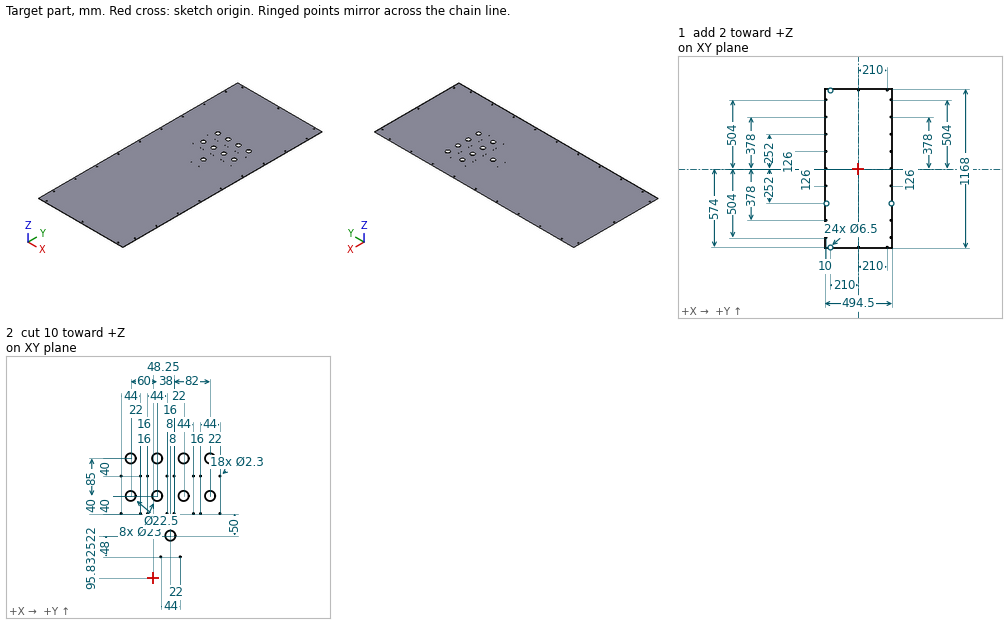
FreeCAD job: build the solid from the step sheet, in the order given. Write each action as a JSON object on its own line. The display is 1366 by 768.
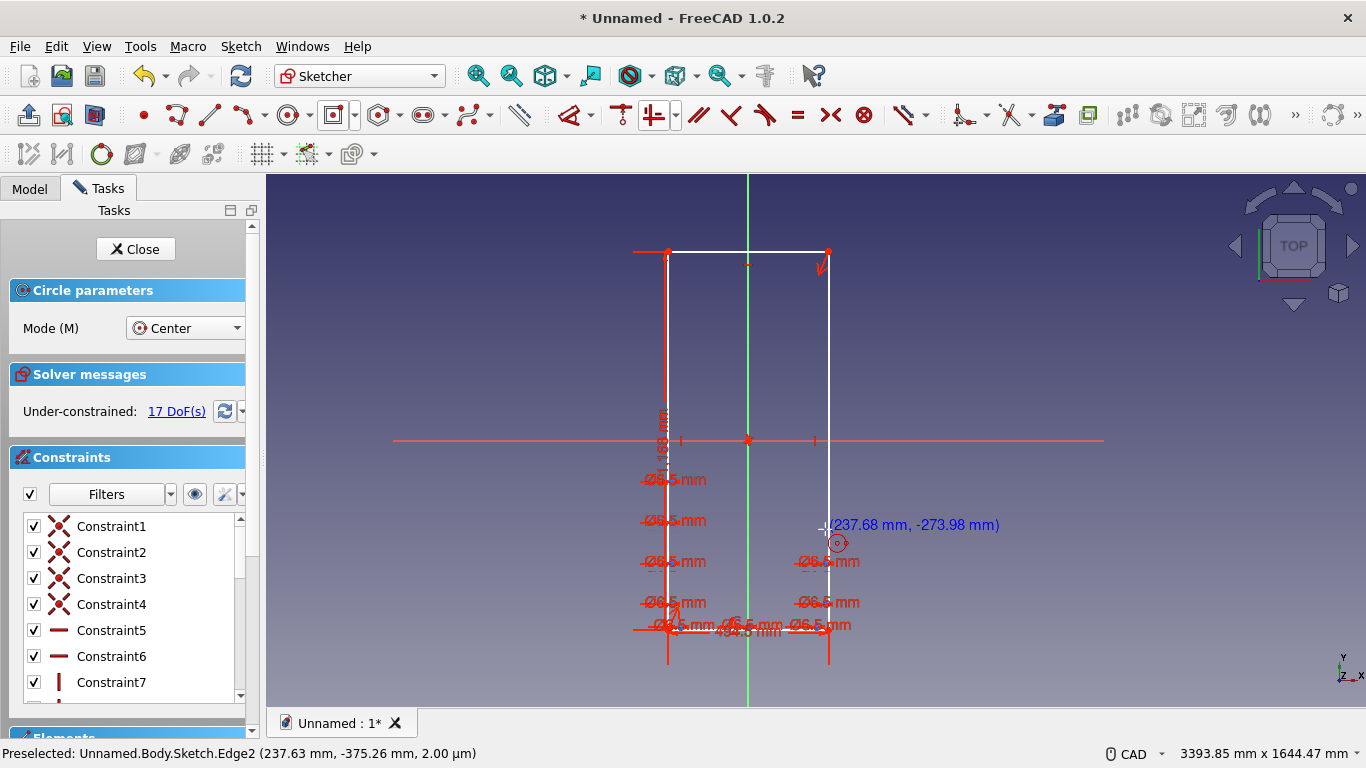
{"action": "scroll", "coordinate": [825, 523], "scroll_direction": "up", "scroll_amount": 8}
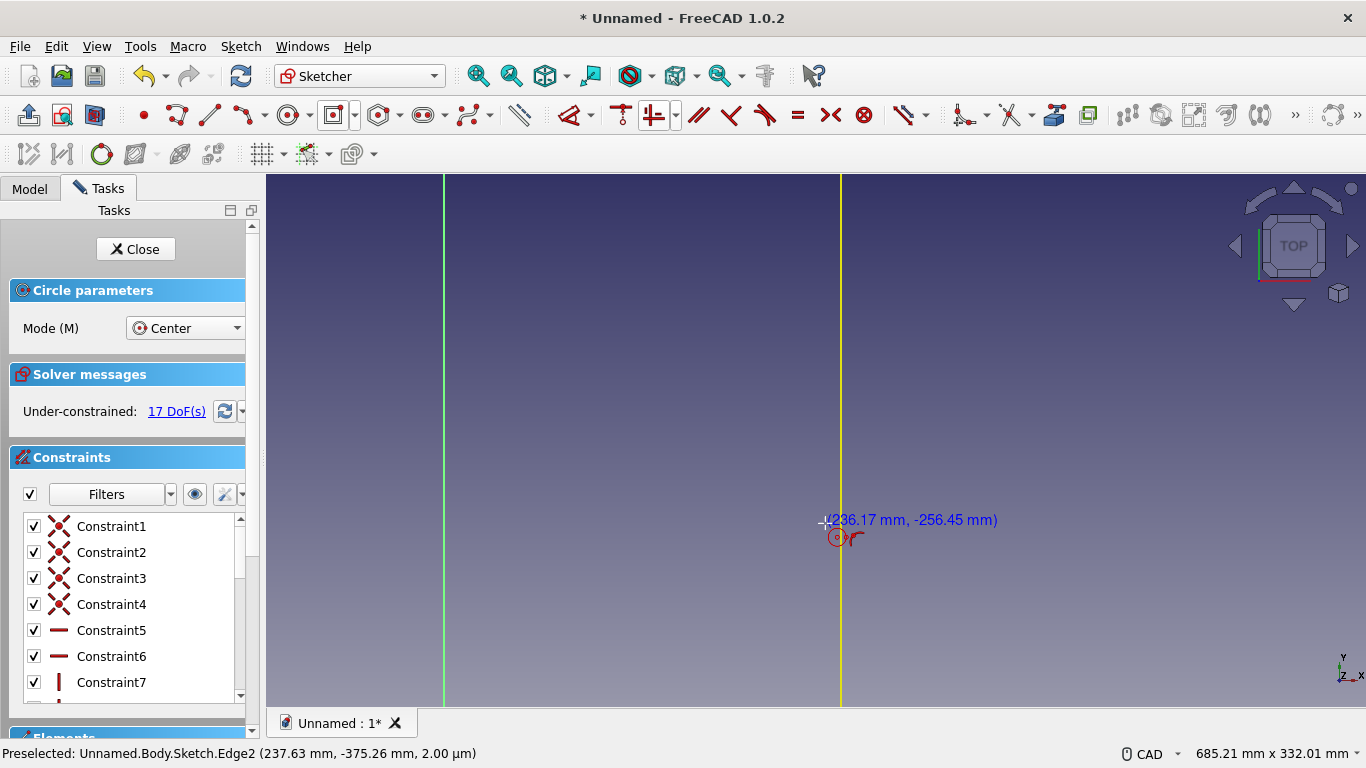
{"action": "left_click", "coordinate": [825, 518]}
{"action": "mouse_move", "coordinate": [821, 515]}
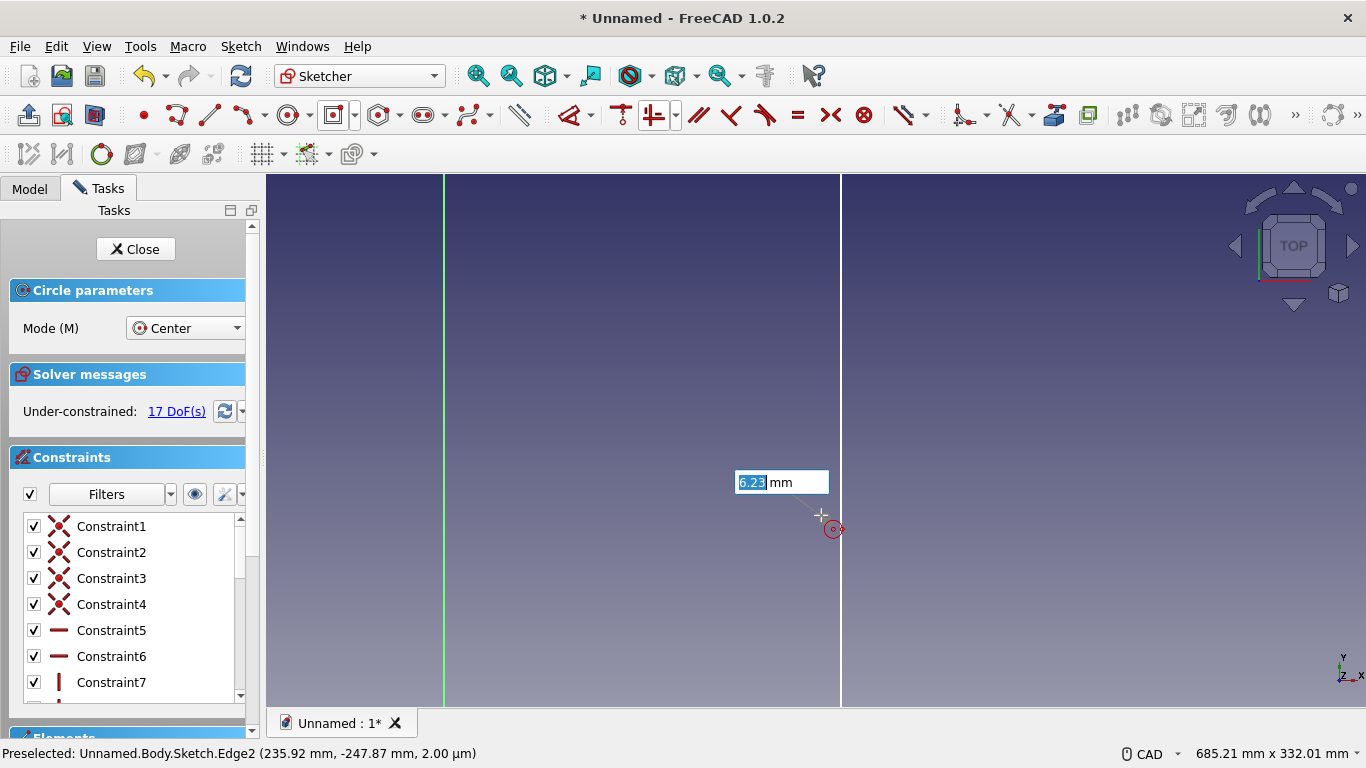
{"action": "type", "text": "6.5"}
{"action": "key", "text": "Return"}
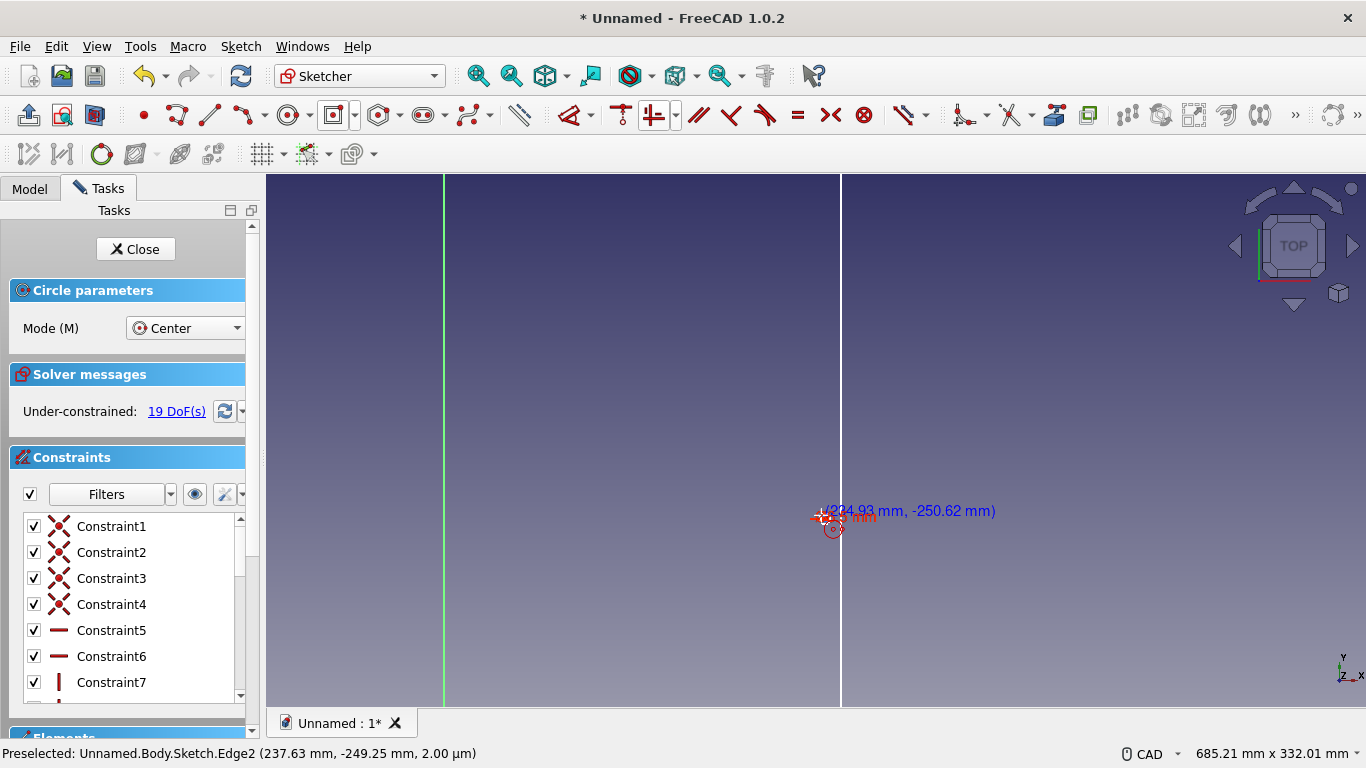
{"action": "scroll", "coordinate": [825, 316], "scroll_direction": "up", "scroll_amount": 8}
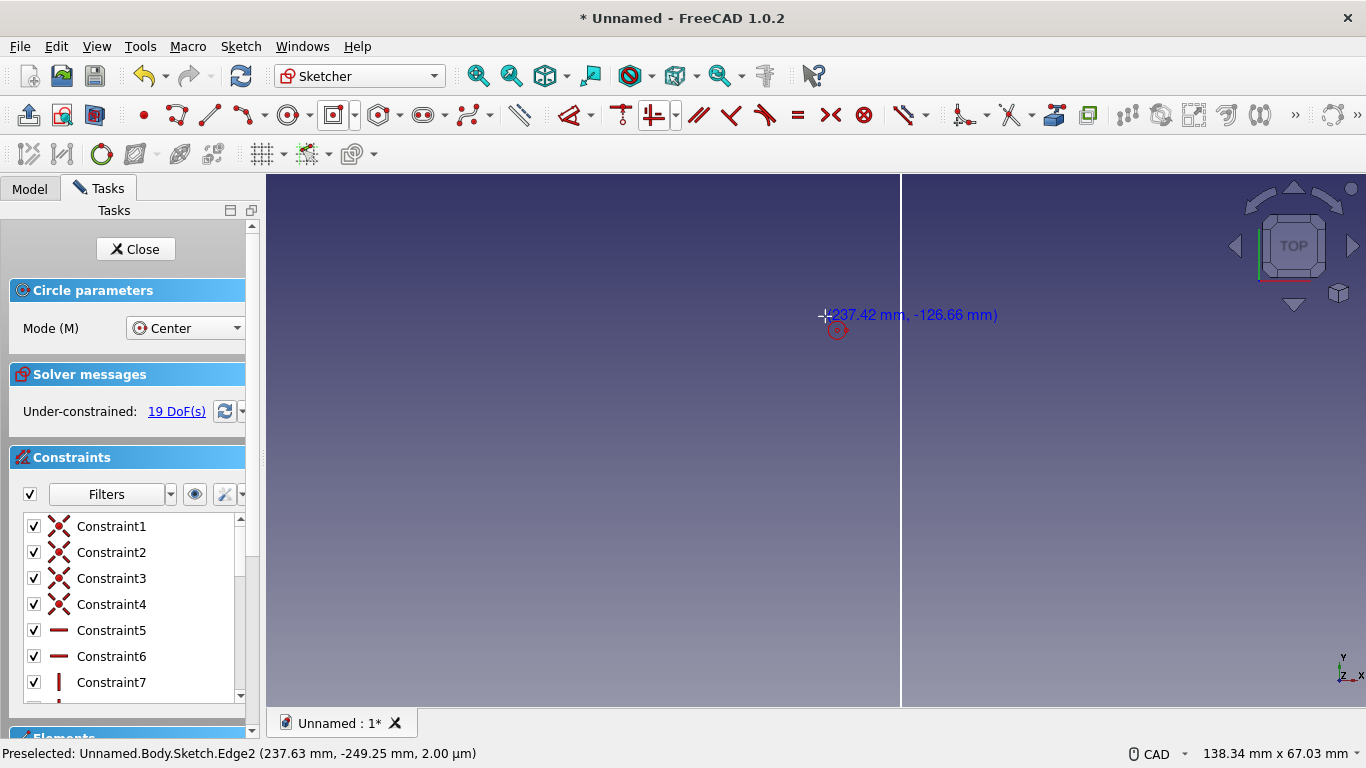
{"action": "scroll", "coordinate": [825, 488], "scroll_direction": "down", "scroll_amount": 16}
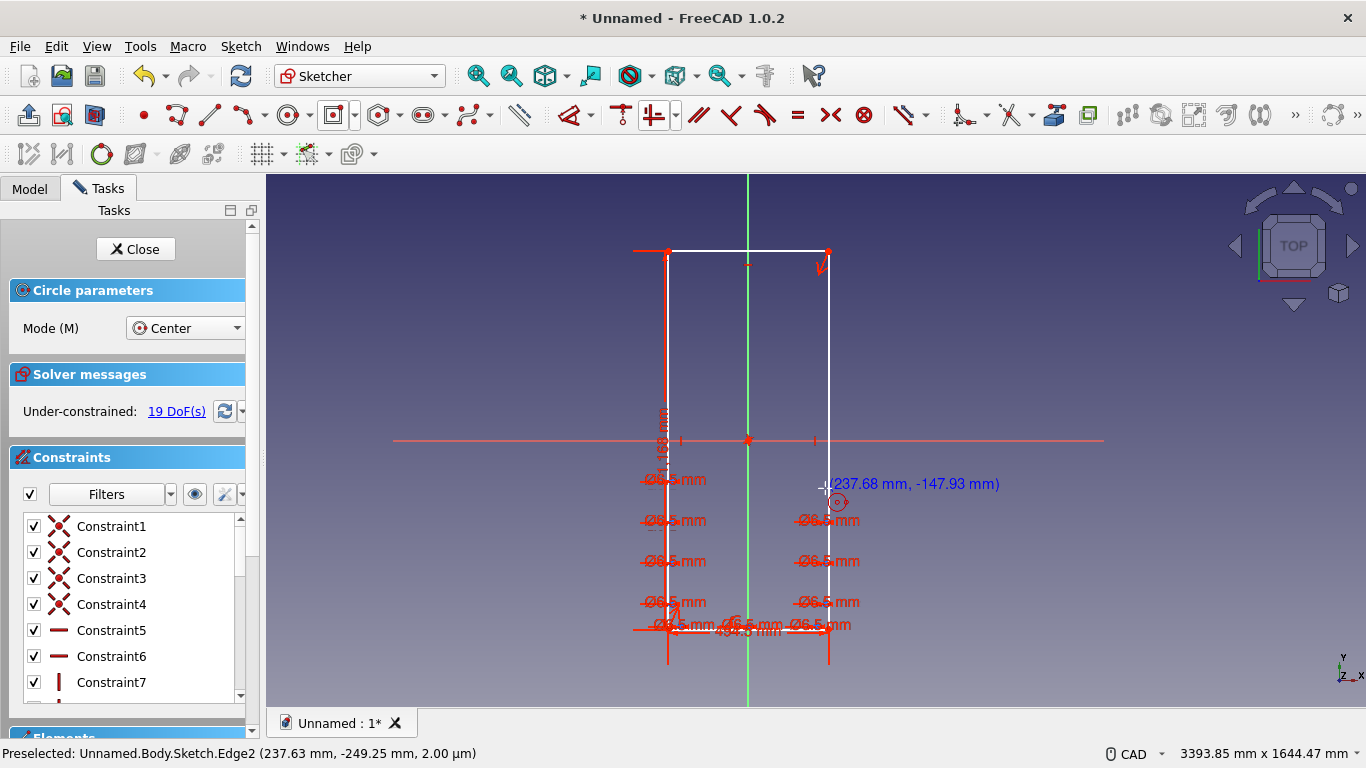
{"action": "scroll", "coordinate": [825, 481], "scroll_direction": "up", "scroll_amount": 8}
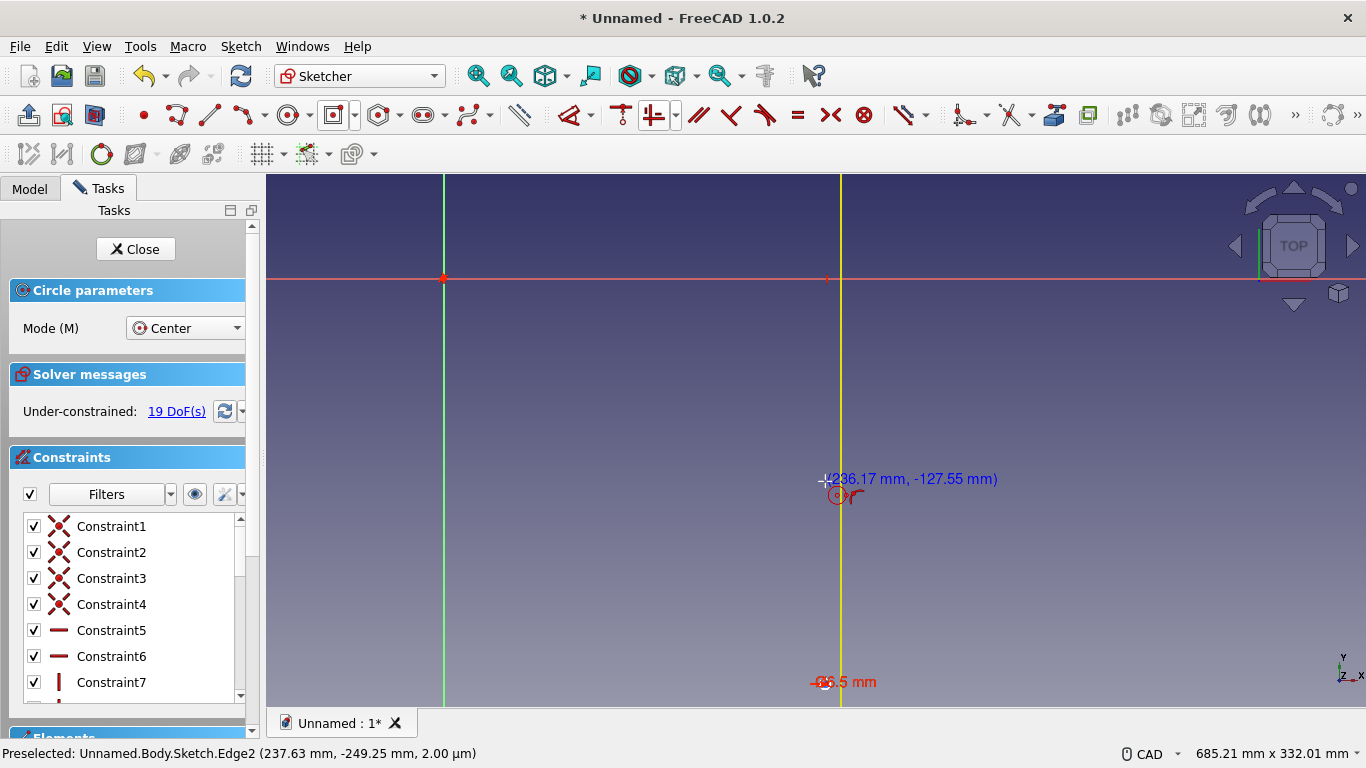
{"action": "left_click", "coordinate": [825, 481]}
{"action": "mouse_move", "coordinate": [821, 477]}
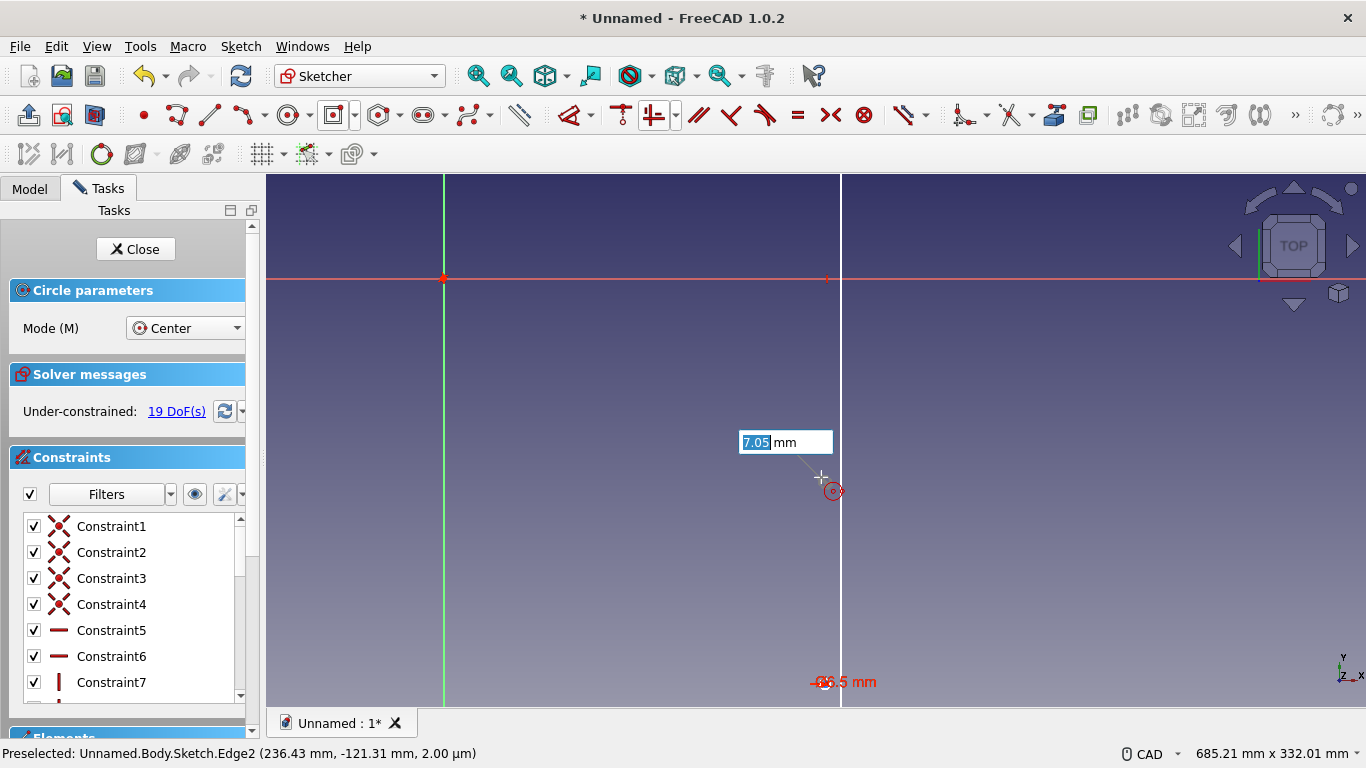
{"action": "type", "text": "6.5"}
{"action": "key", "text": "Return"}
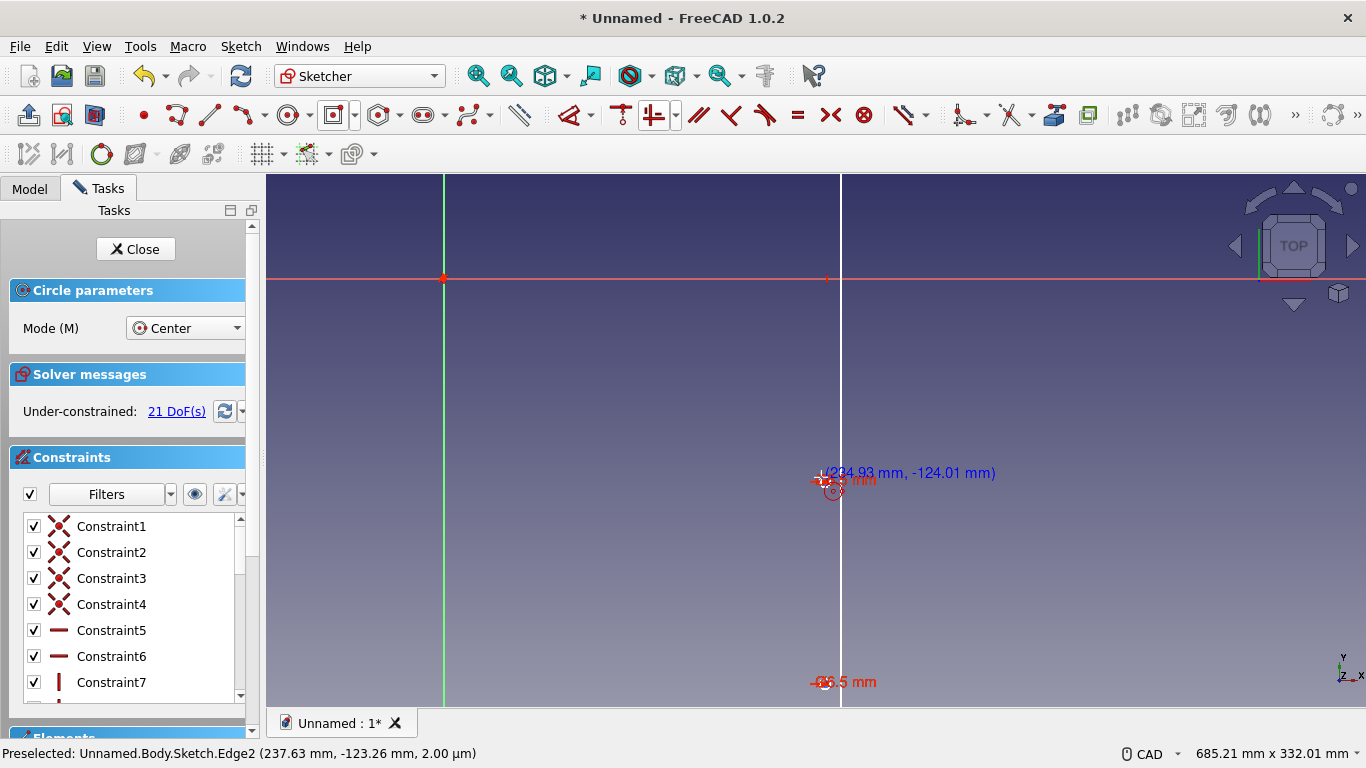
{"action": "scroll", "coordinate": [808, 472], "scroll_direction": "down", "scroll_amount": 9}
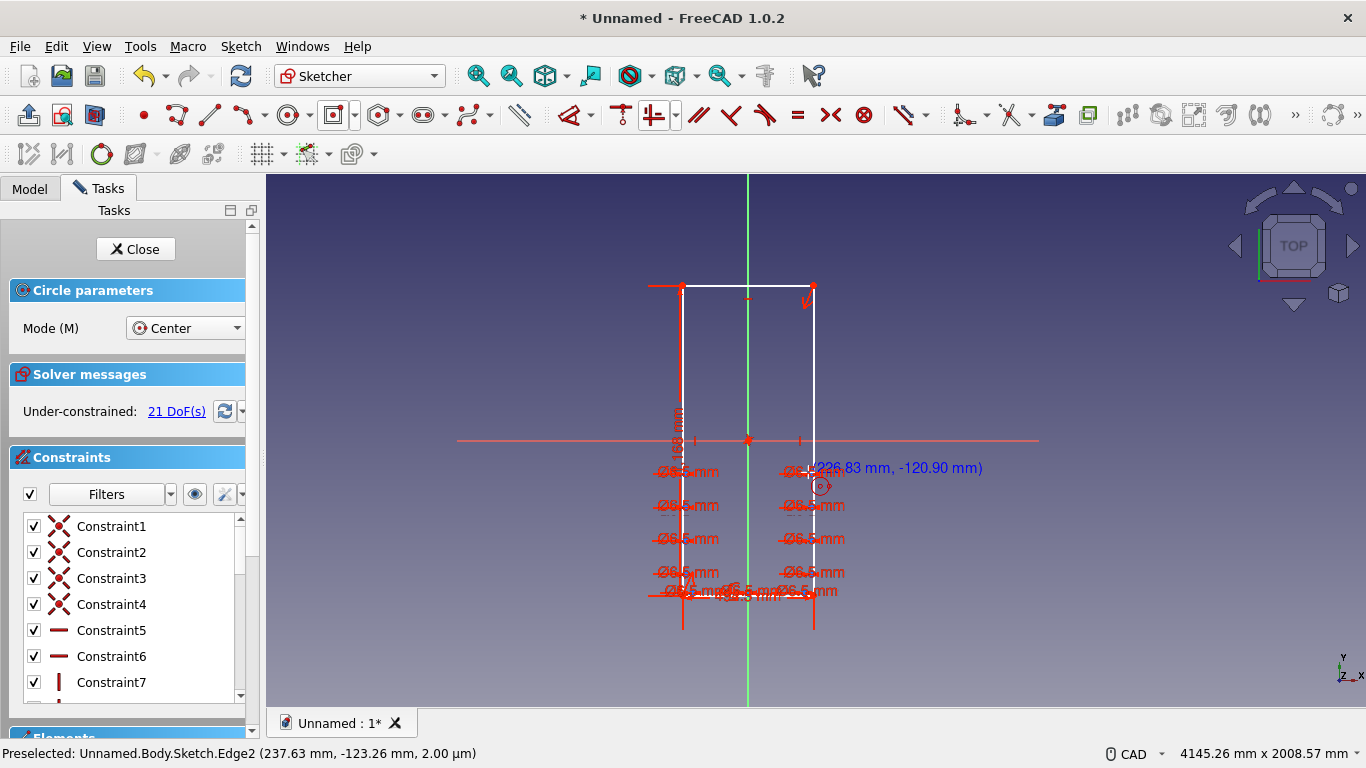
{"action": "scroll", "coordinate": [685, 441], "scroll_direction": "up", "scroll_amount": 17}